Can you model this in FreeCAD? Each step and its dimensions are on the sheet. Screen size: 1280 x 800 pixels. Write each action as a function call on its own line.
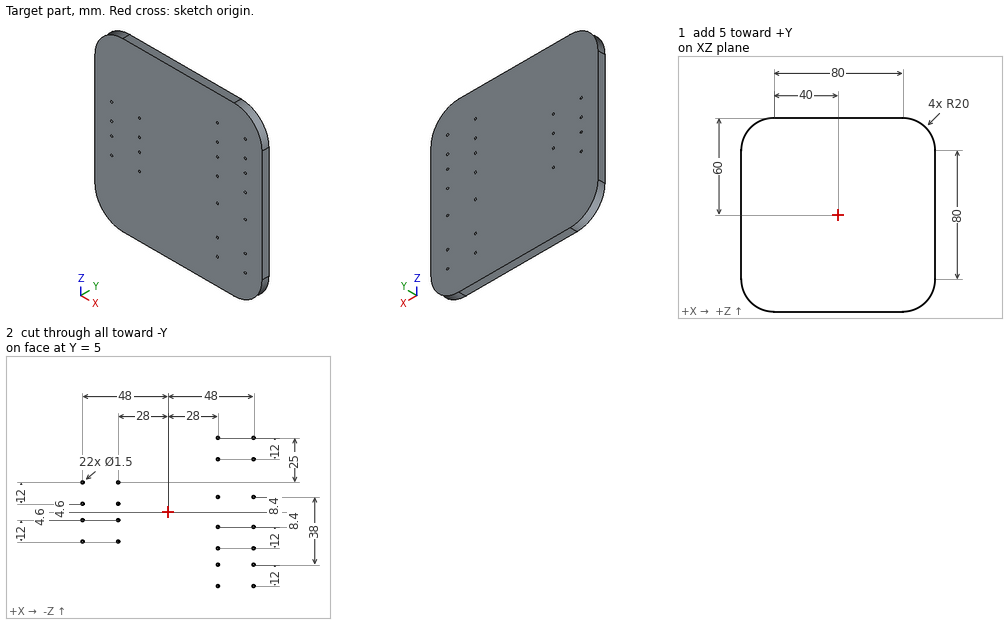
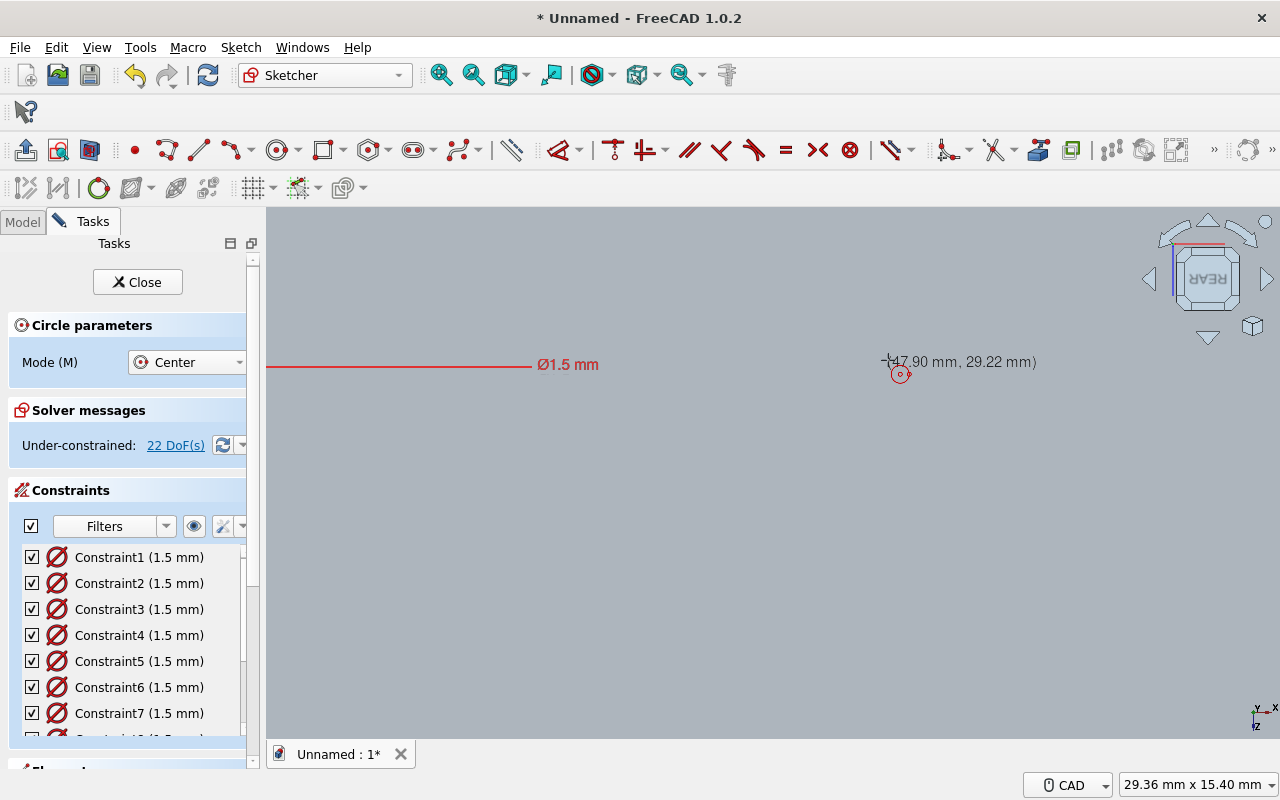
scroll(888, 360, down, 11)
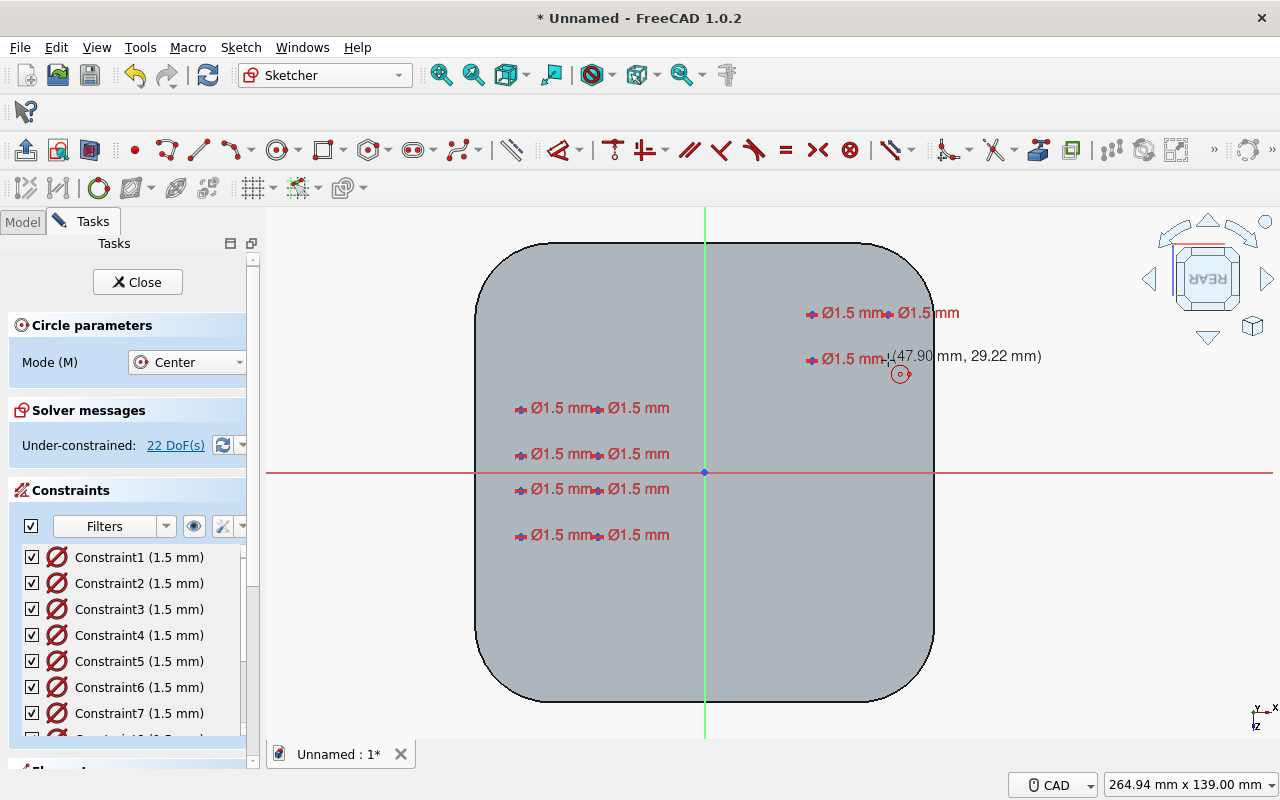
click(888, 360)
move(890, 358)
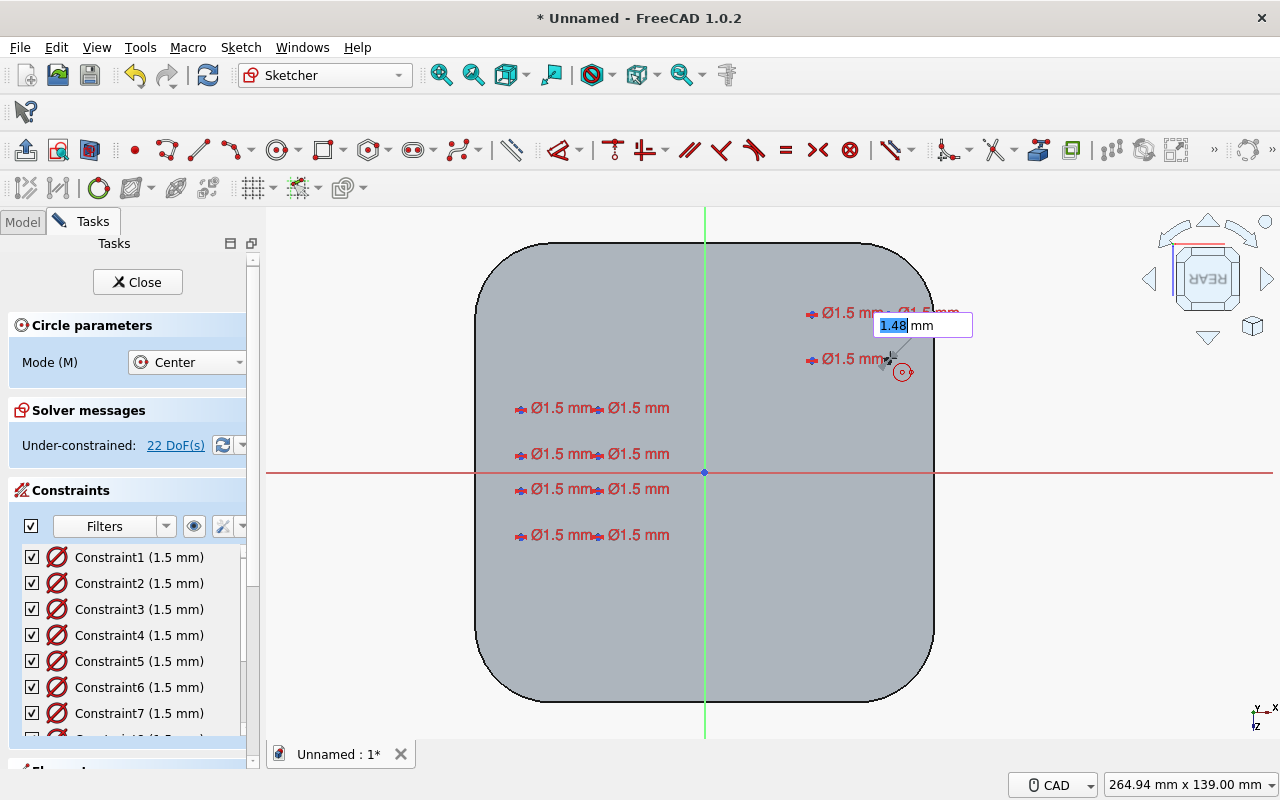
text(1.5)
key(Return)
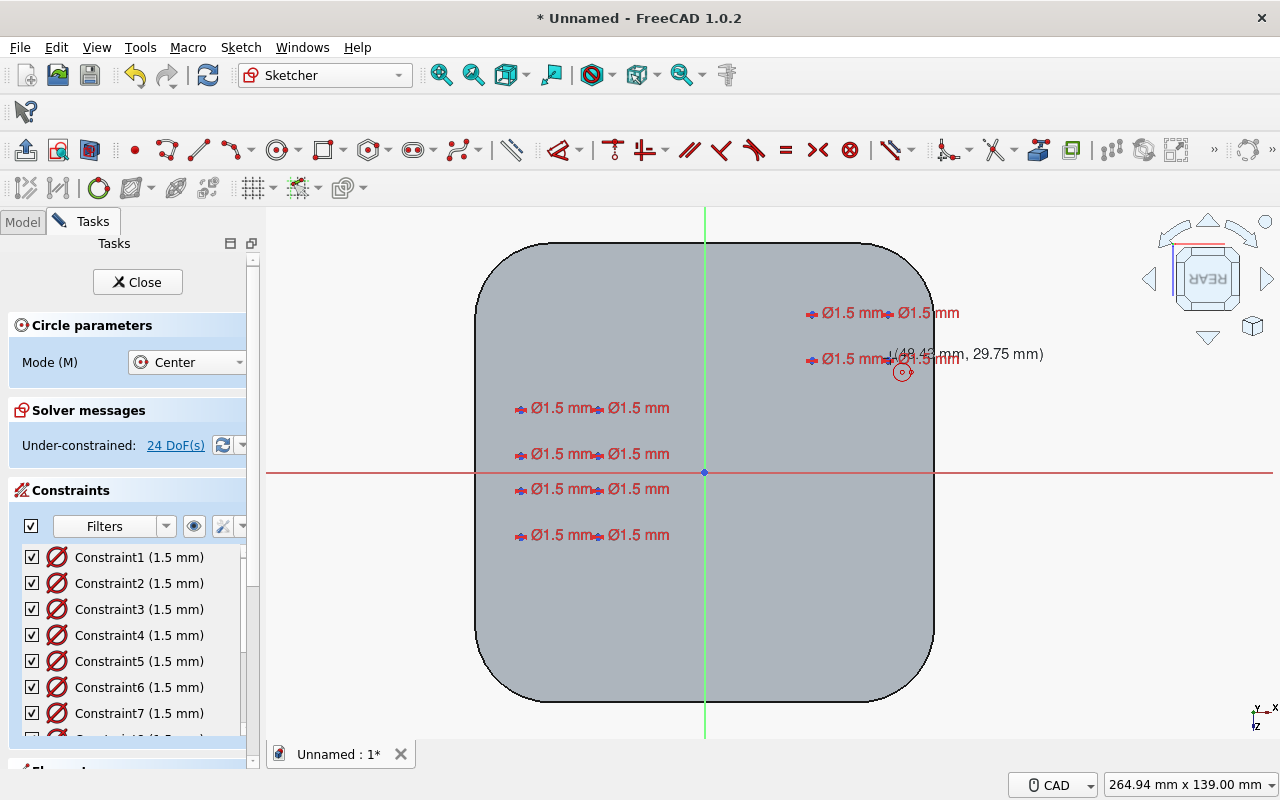
scroll(888, 441, up, 11)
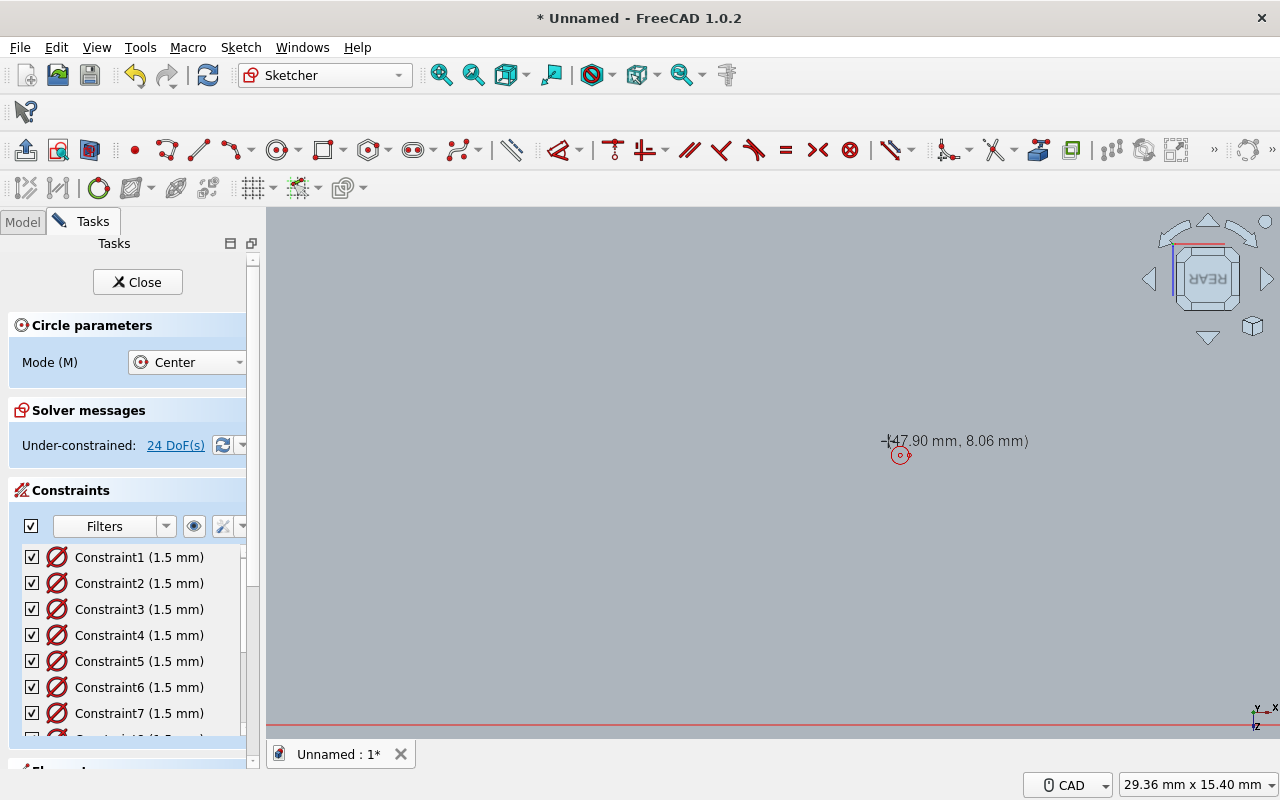
scroll(888, 442, down, 11)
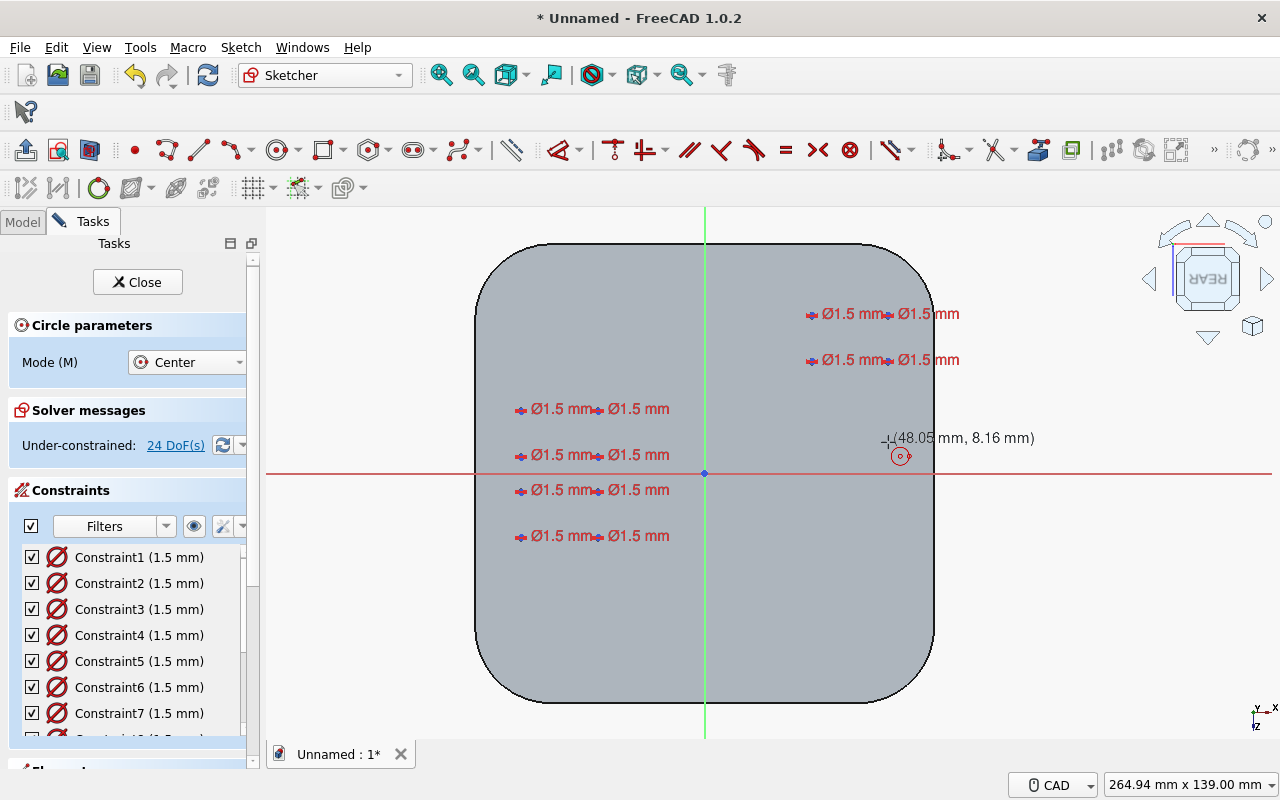
click(888, 442)
move(890, 440)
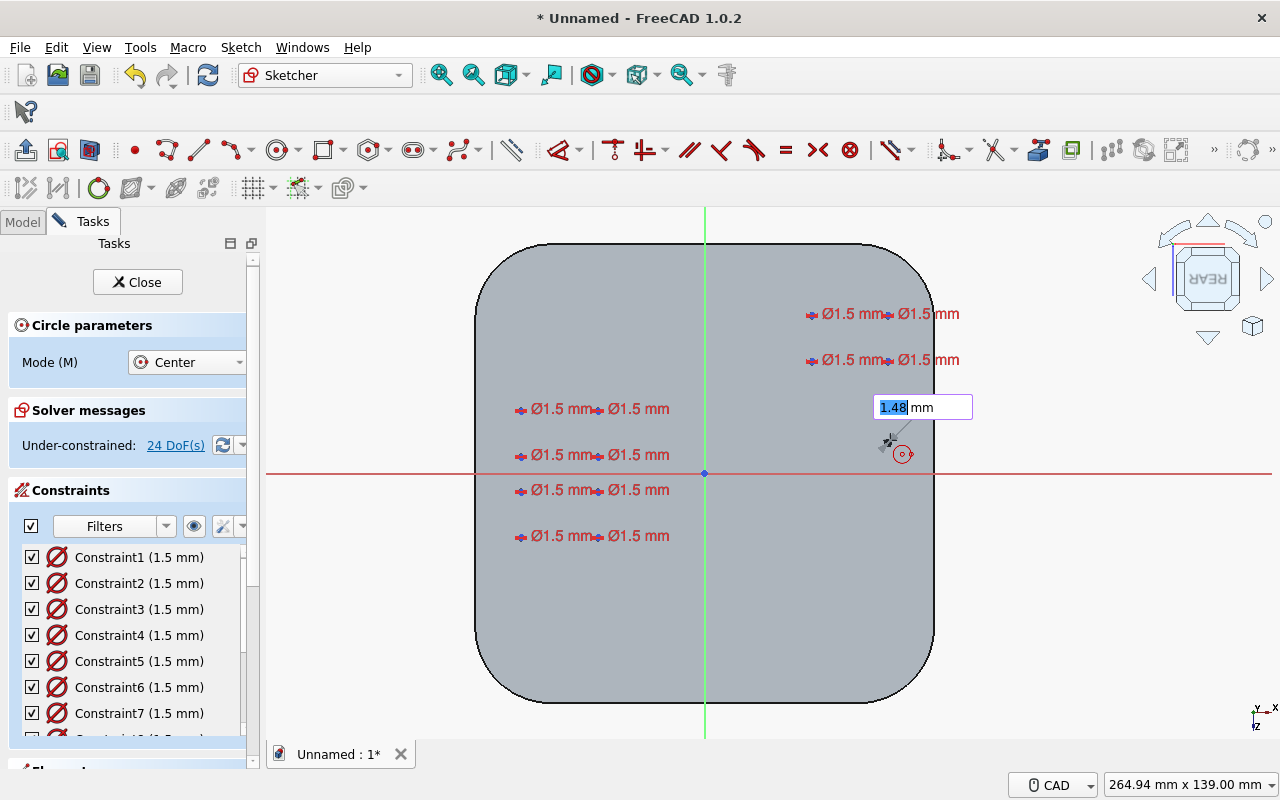
text(1.5)
key(Return)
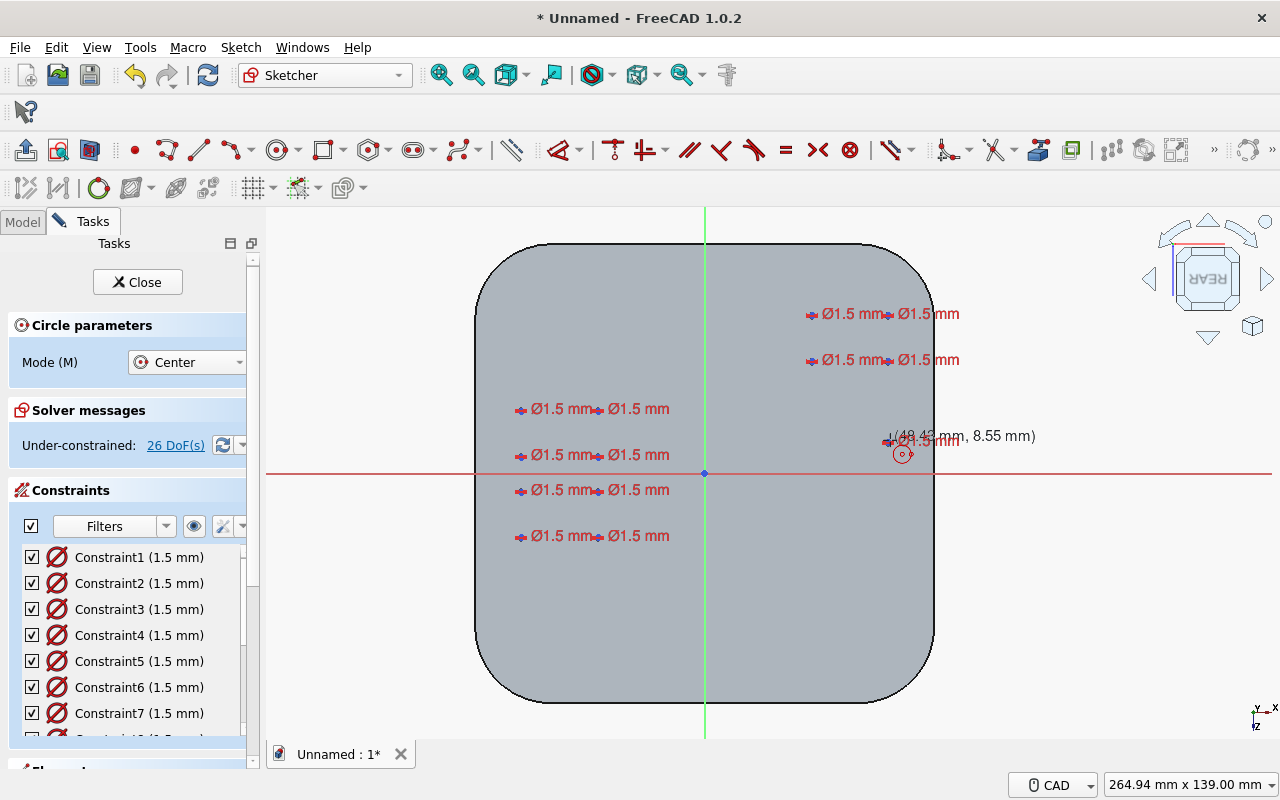
scroll(812, 442, up, 11)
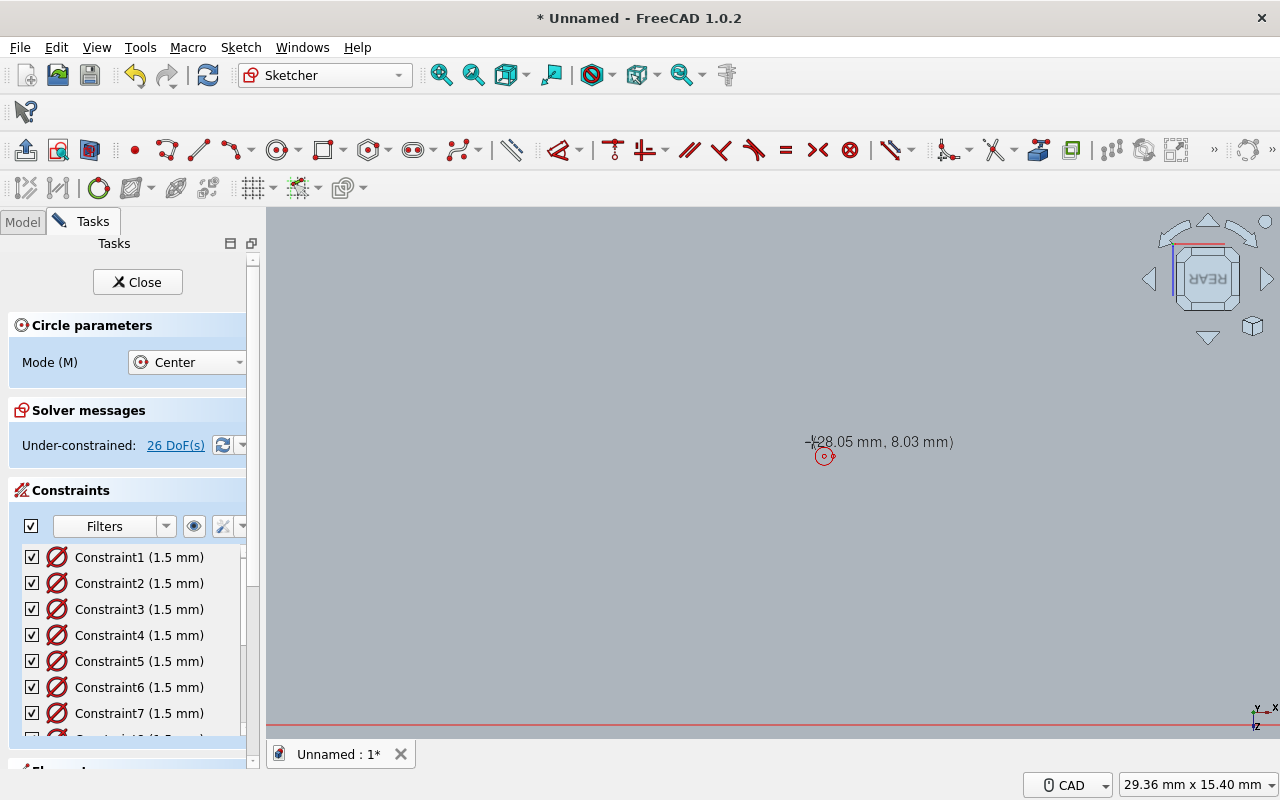
scroll(812, 442, down, 11)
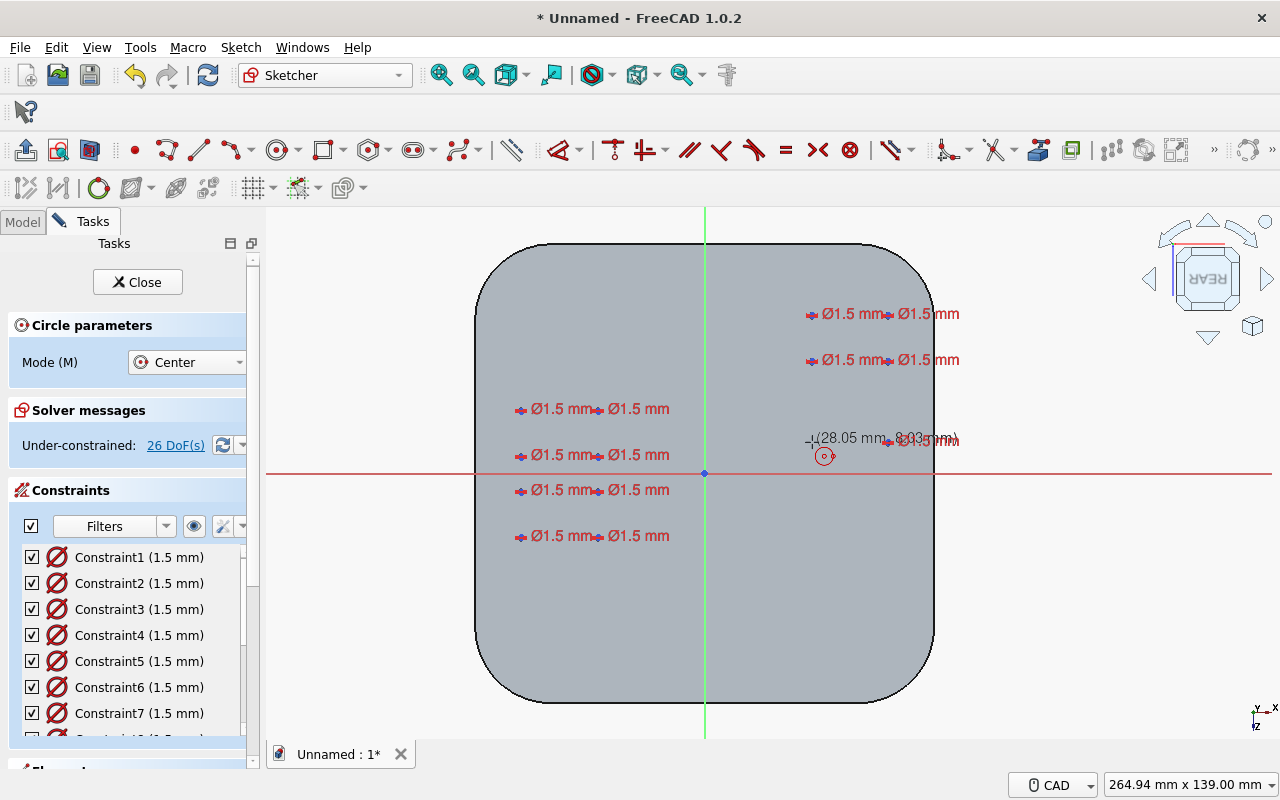
click(812, 442)
move(814, 440)